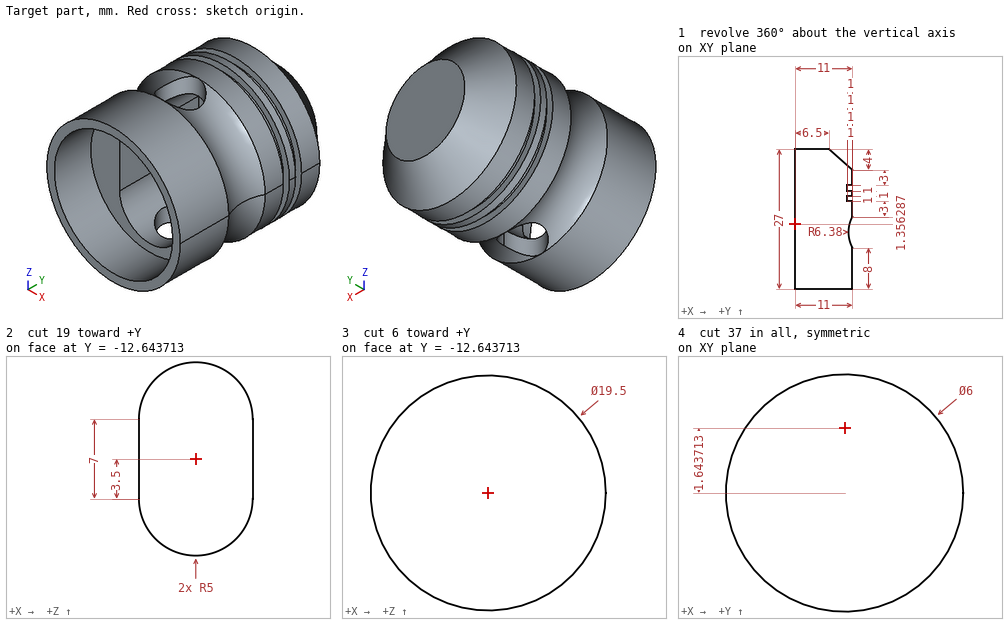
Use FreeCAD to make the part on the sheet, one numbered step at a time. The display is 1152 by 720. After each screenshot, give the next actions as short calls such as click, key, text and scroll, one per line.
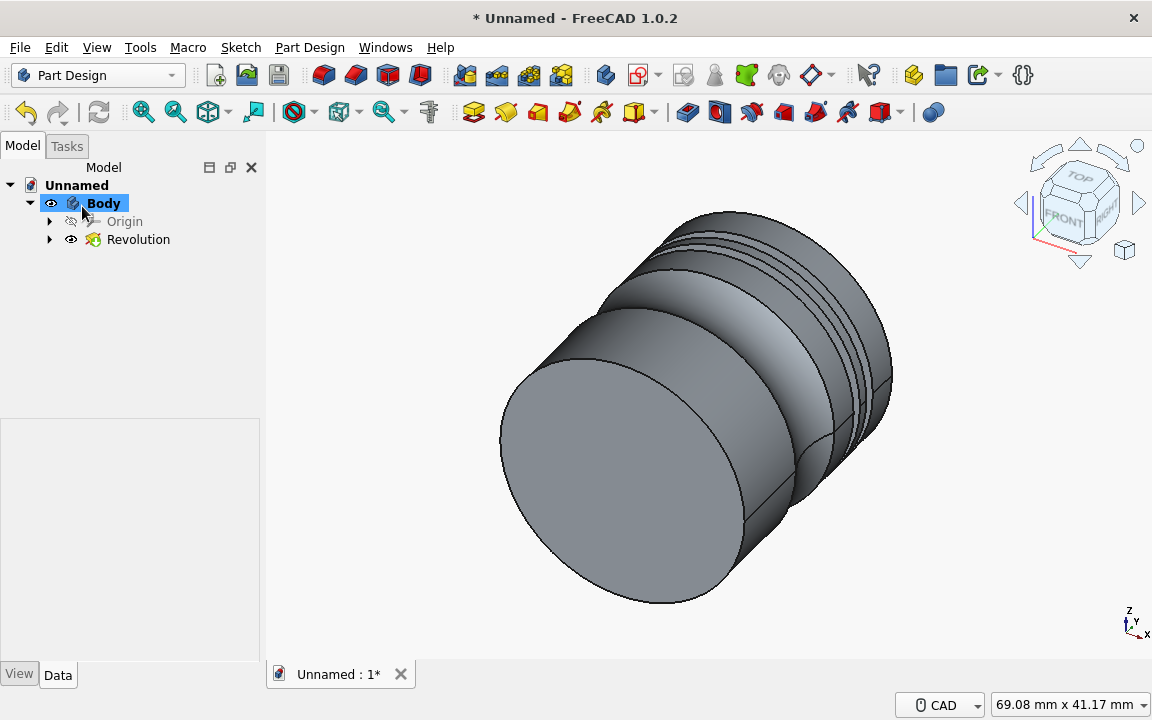
click(622, 480)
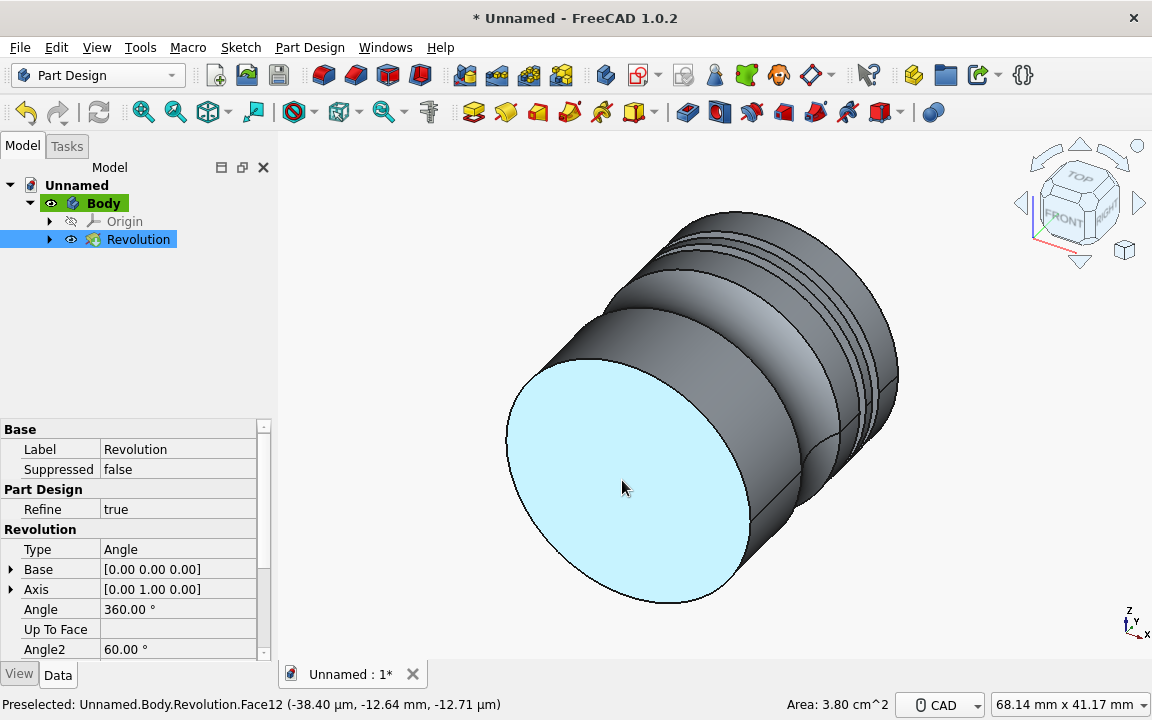
click(638, 76)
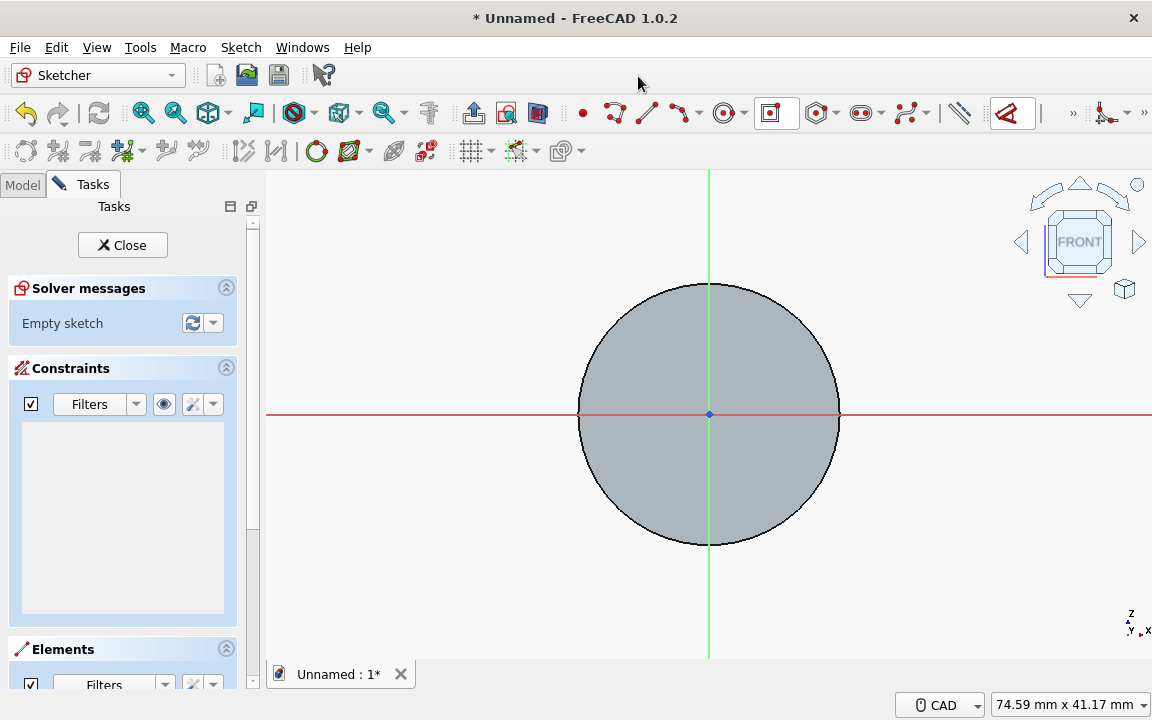
scroll(848, 414, up, 2)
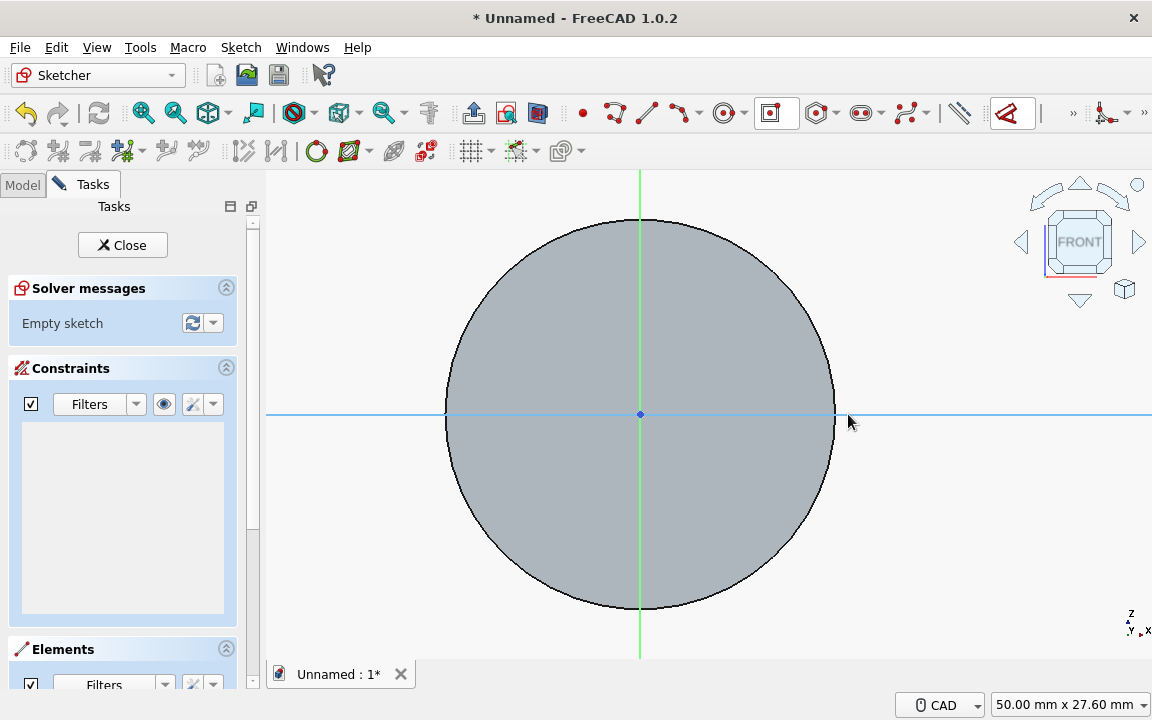
click(862, 114)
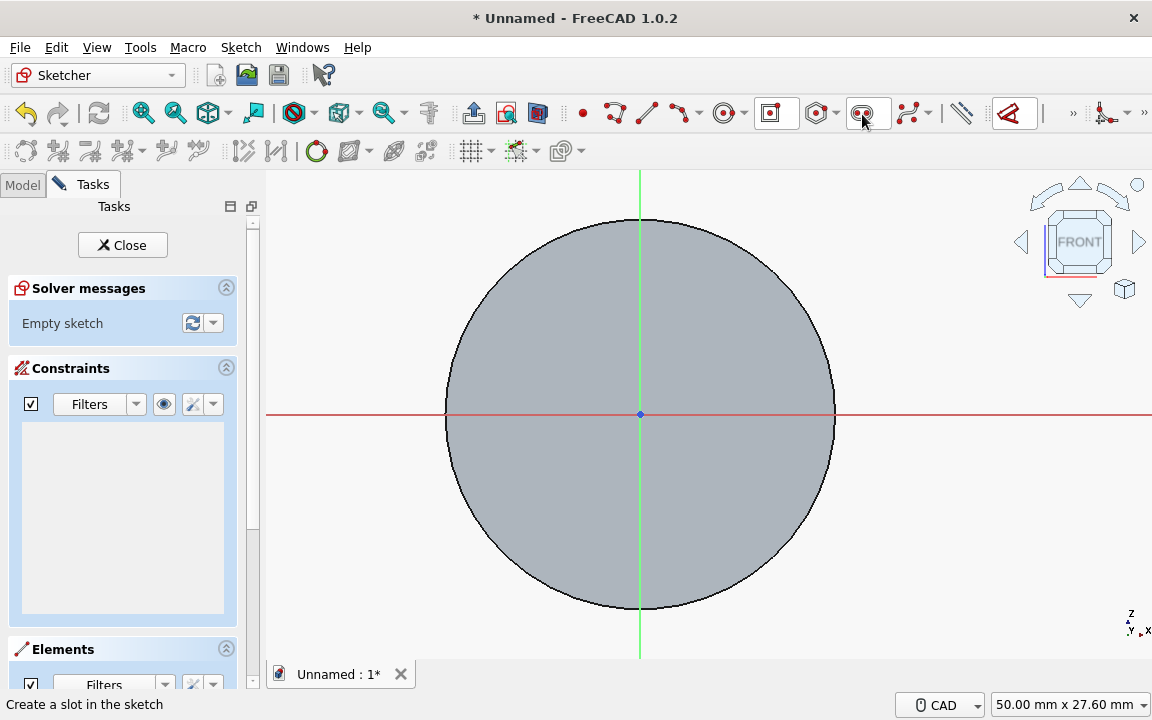
click(640, 477)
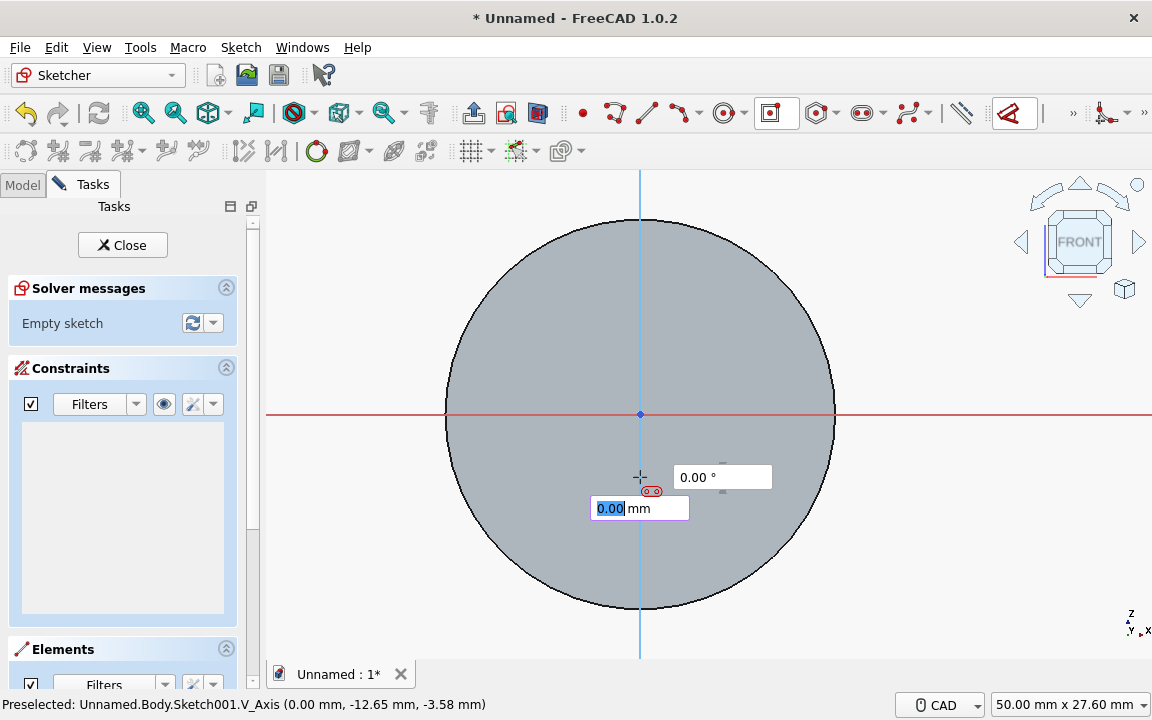
click(649, 352)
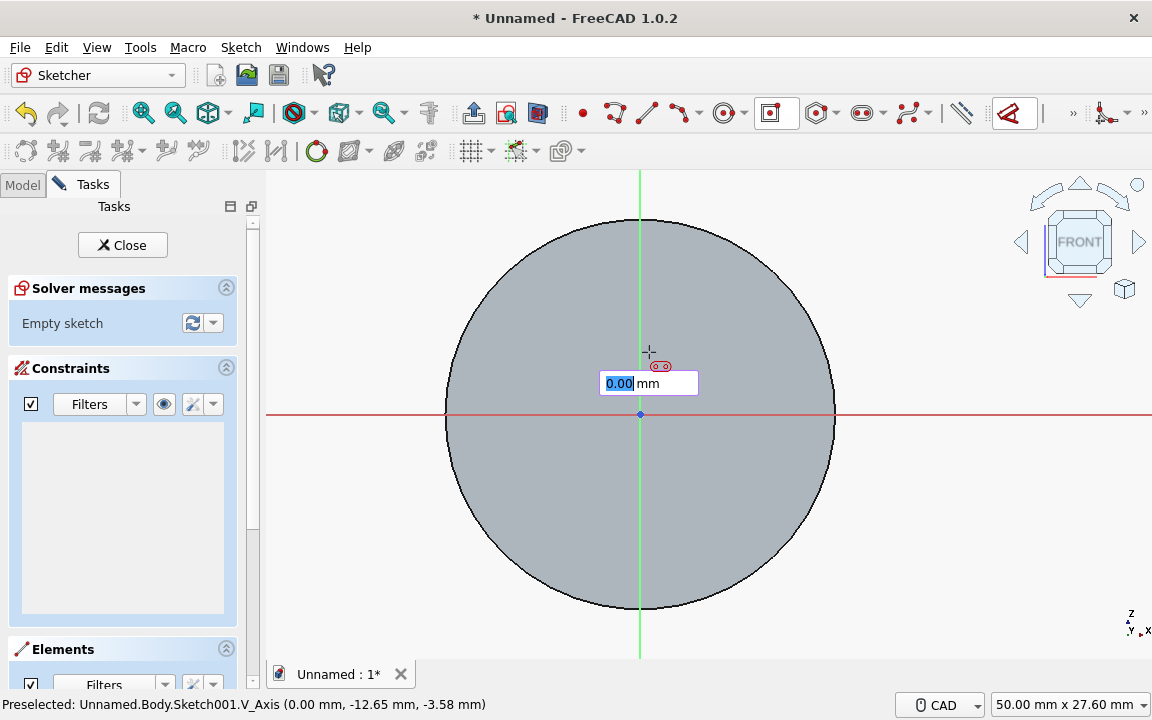
click(552, 396)
key(Escape)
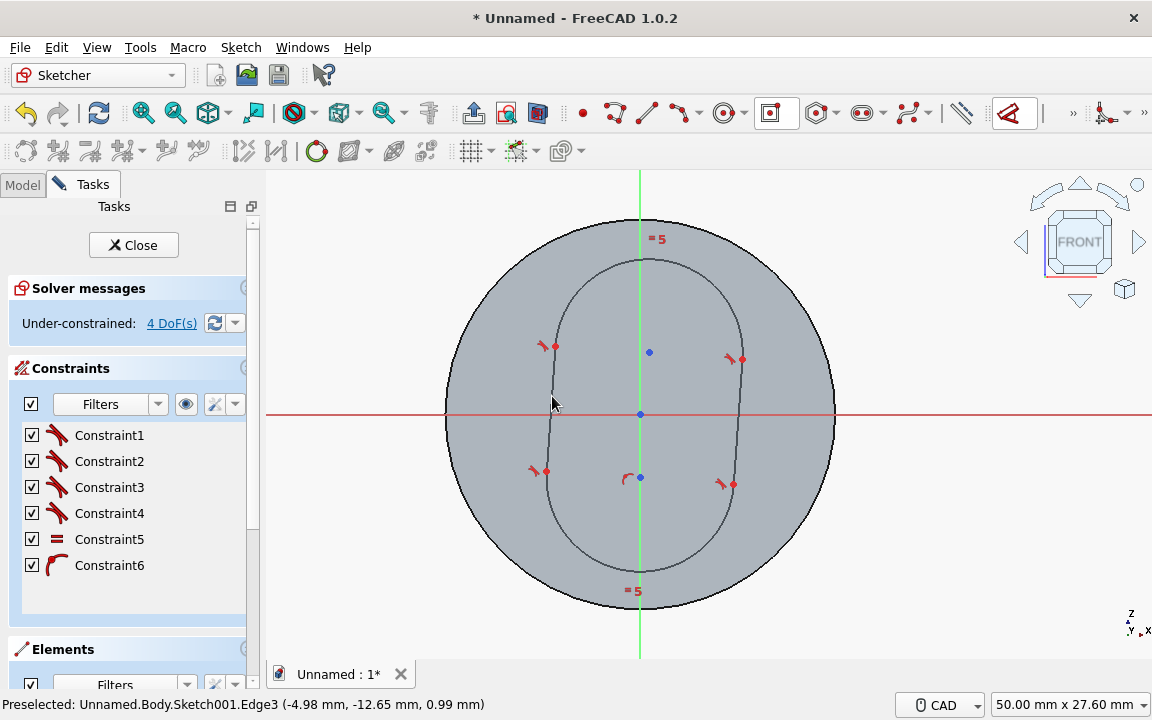
click(549, 434)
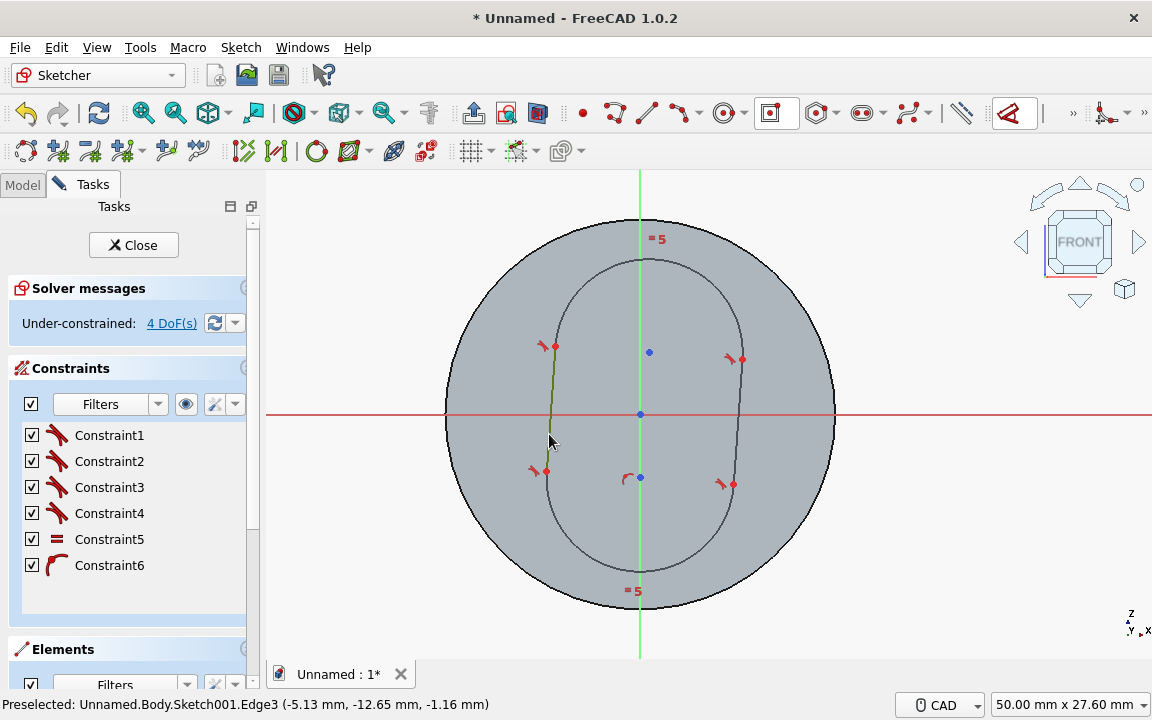
key(v)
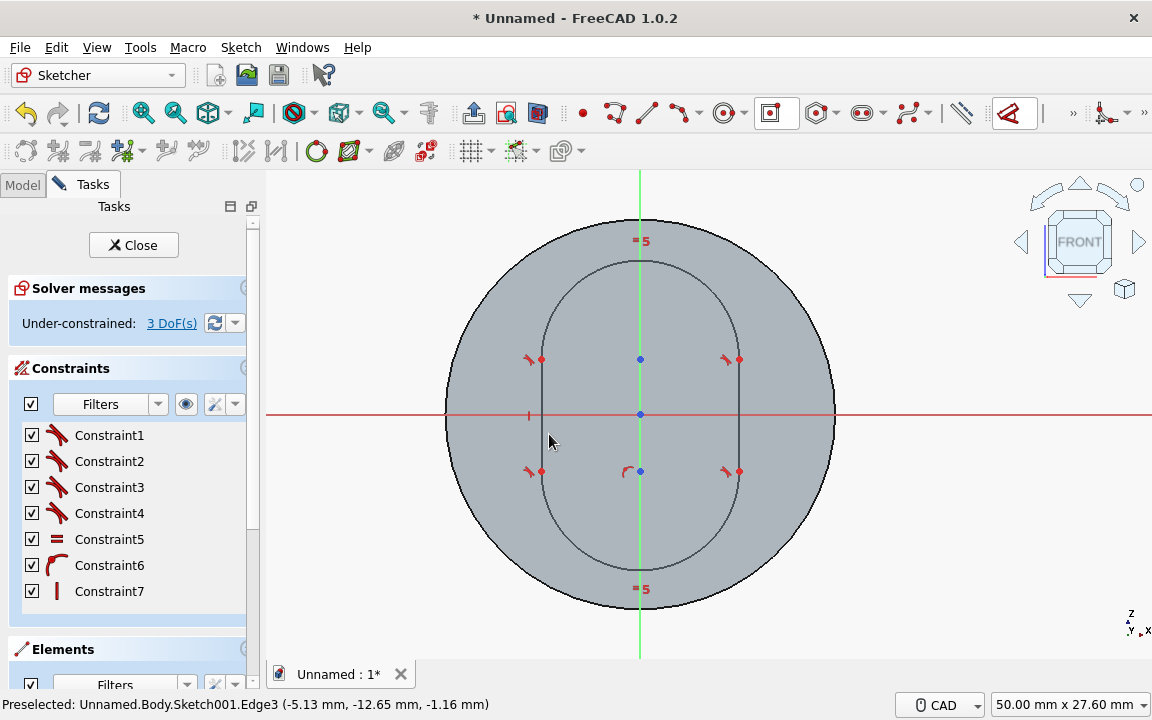
click(582, 551)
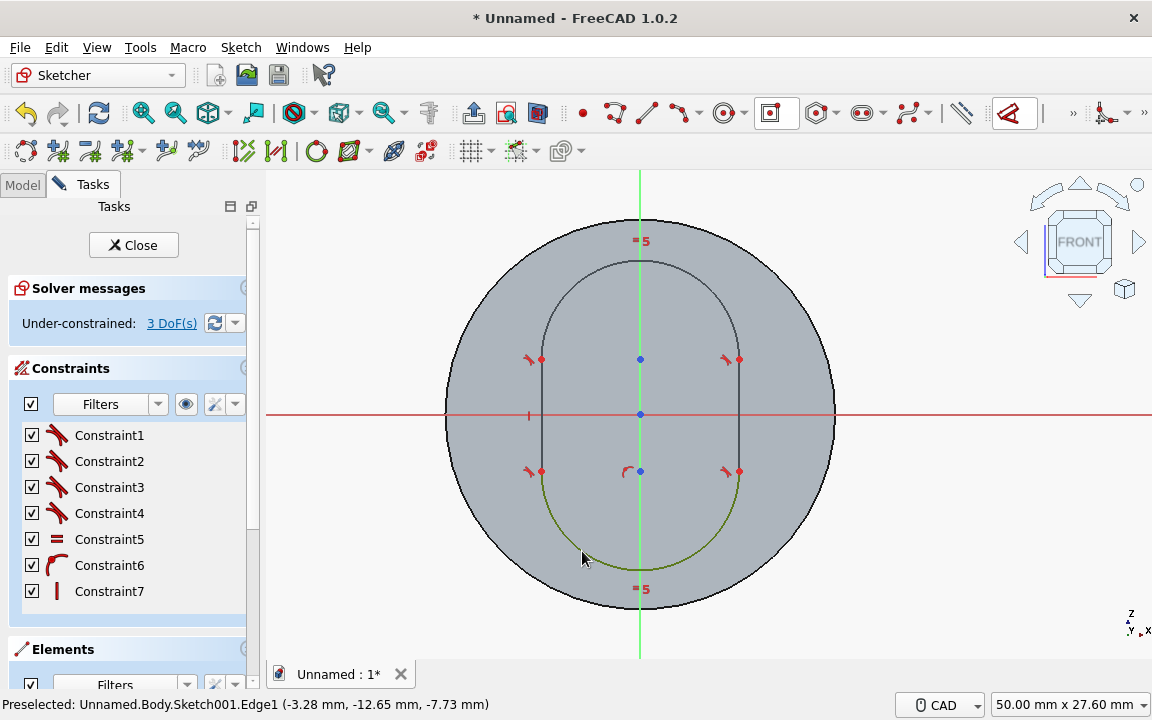
click(1032, 114)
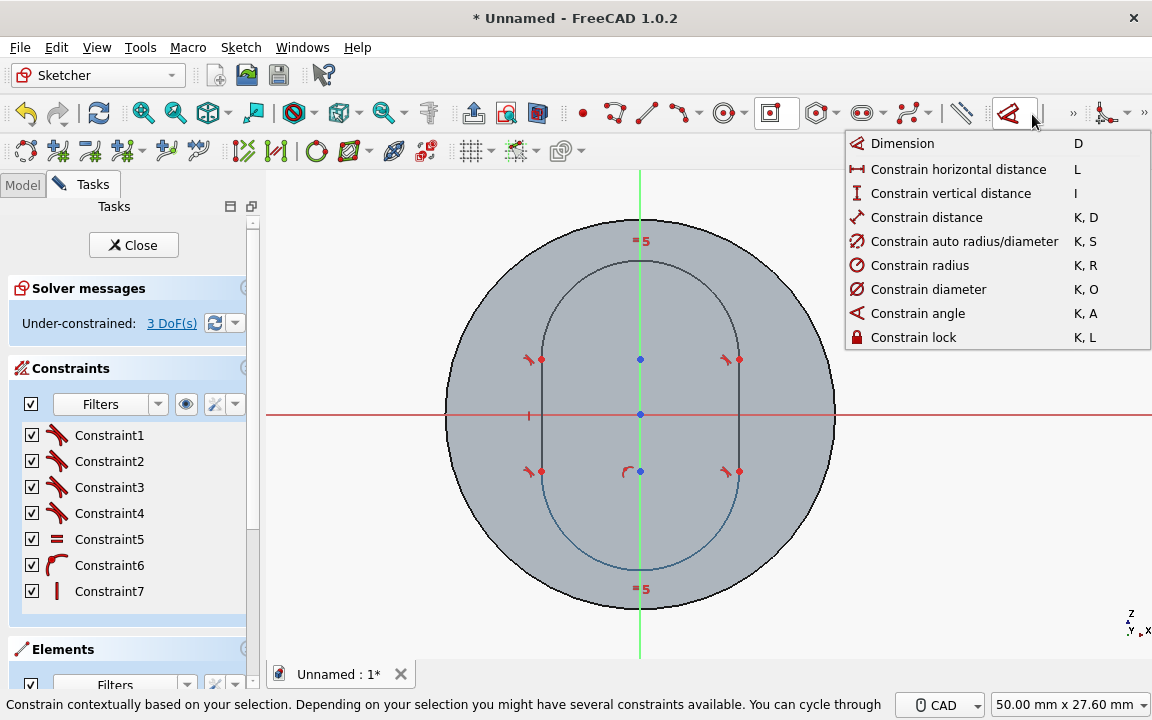
click(998, 265)